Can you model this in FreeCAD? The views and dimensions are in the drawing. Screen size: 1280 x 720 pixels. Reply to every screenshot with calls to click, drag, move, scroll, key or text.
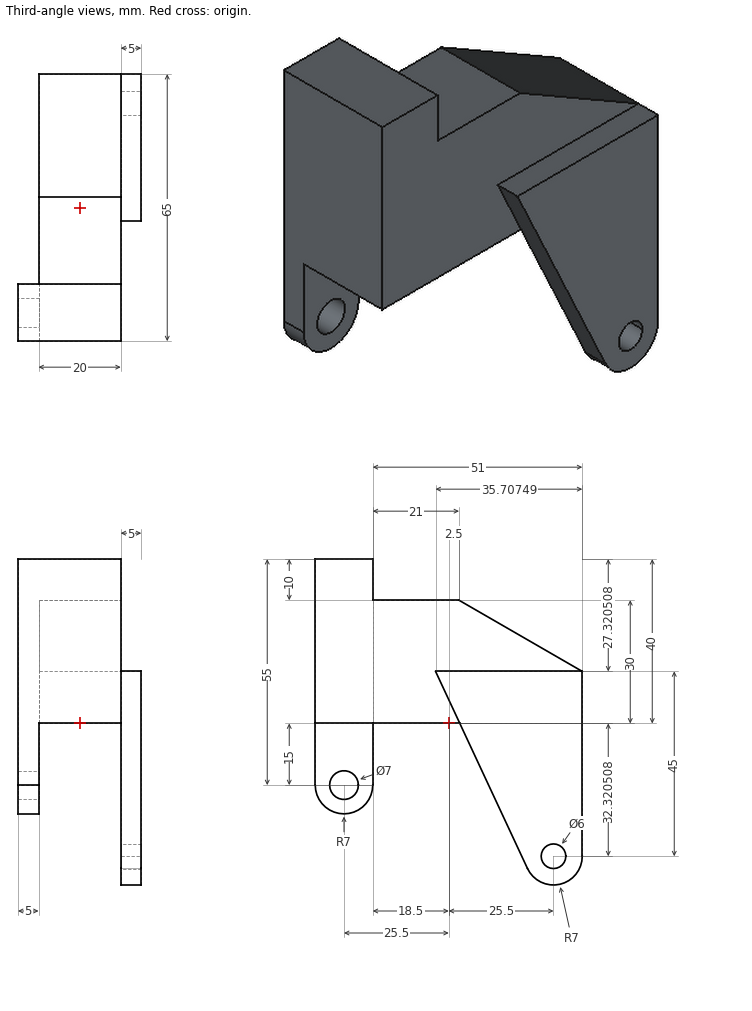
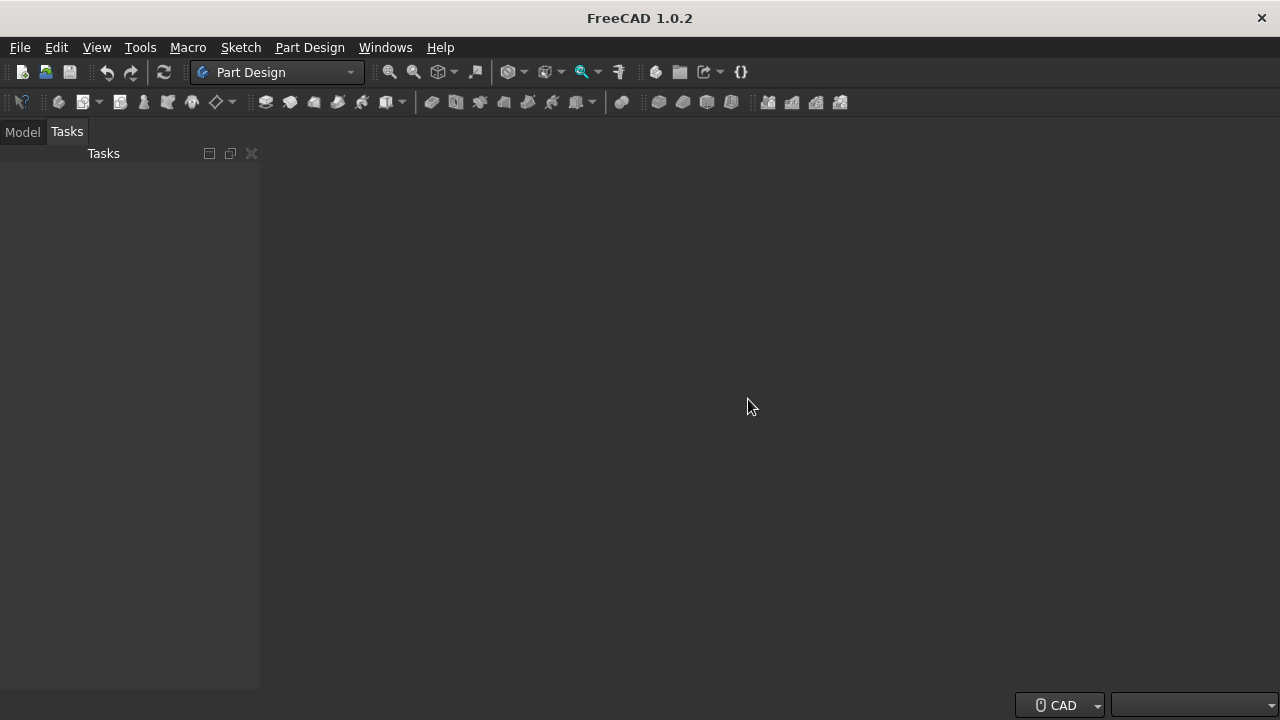
key(ctrl+n)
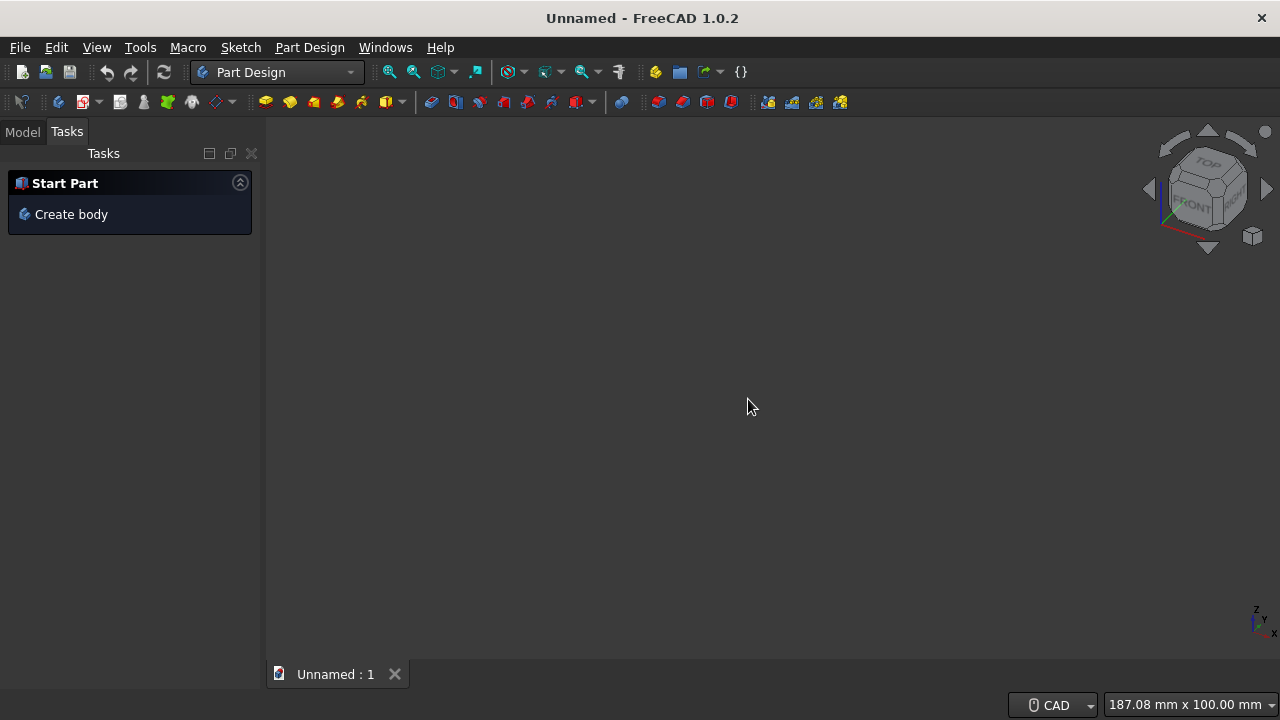
click(84, 102)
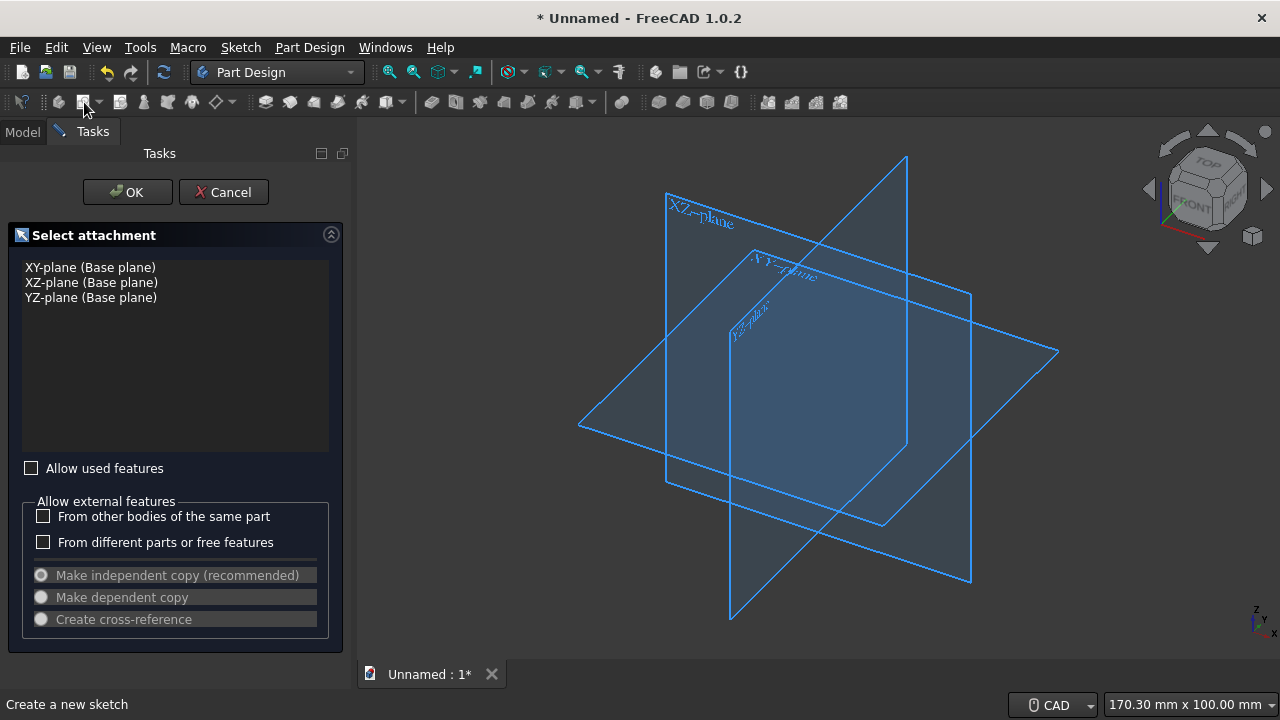
click(82, 268)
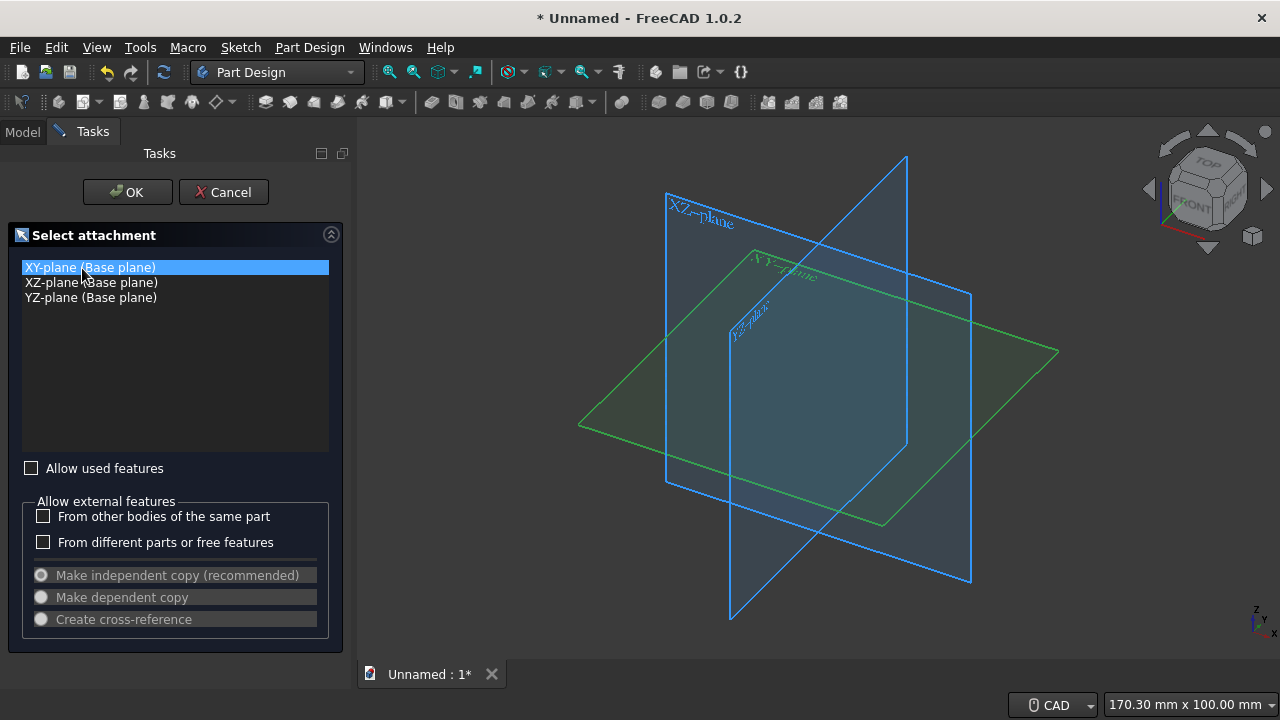
click(128, 192)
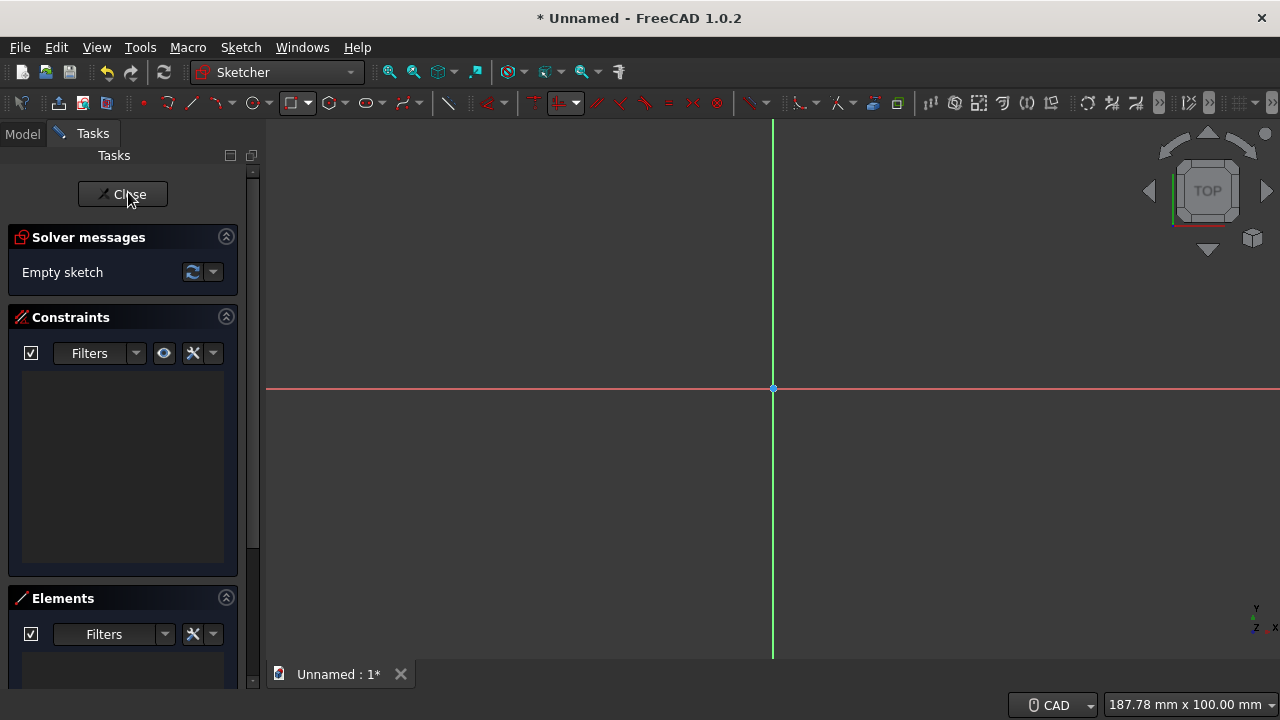
key(g)
key(v)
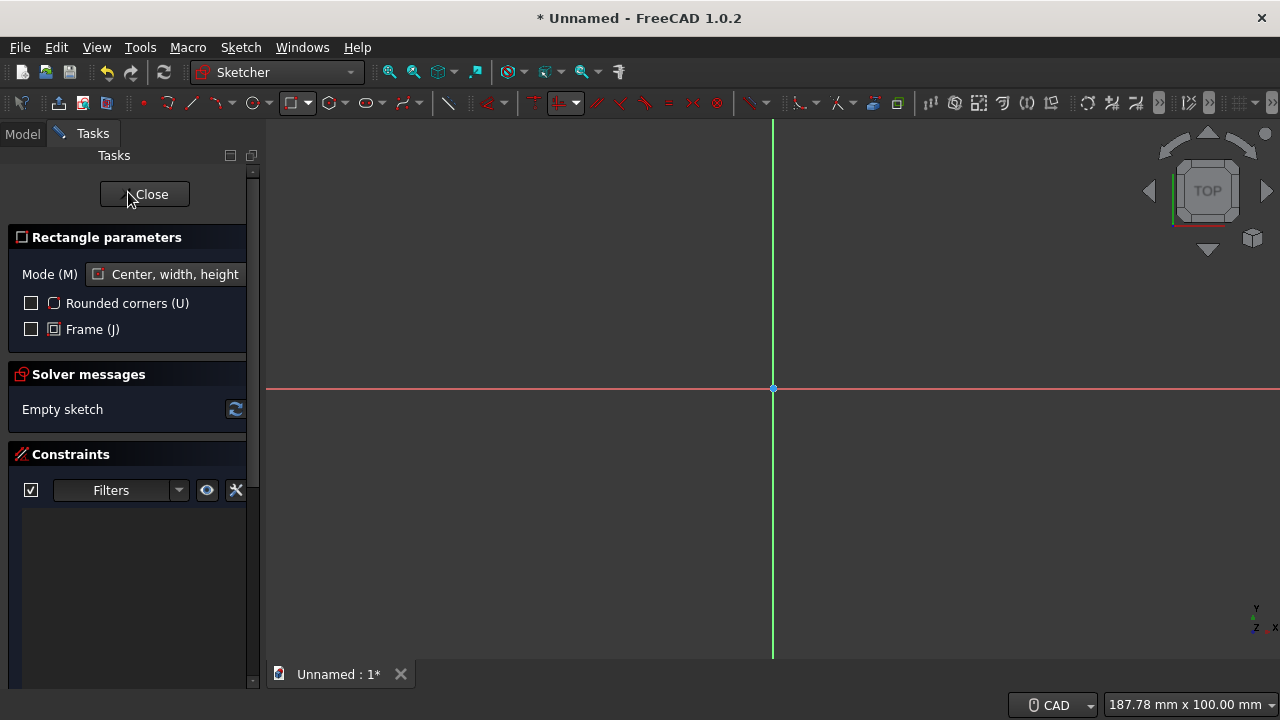
click(773, 389)
move(827, 214)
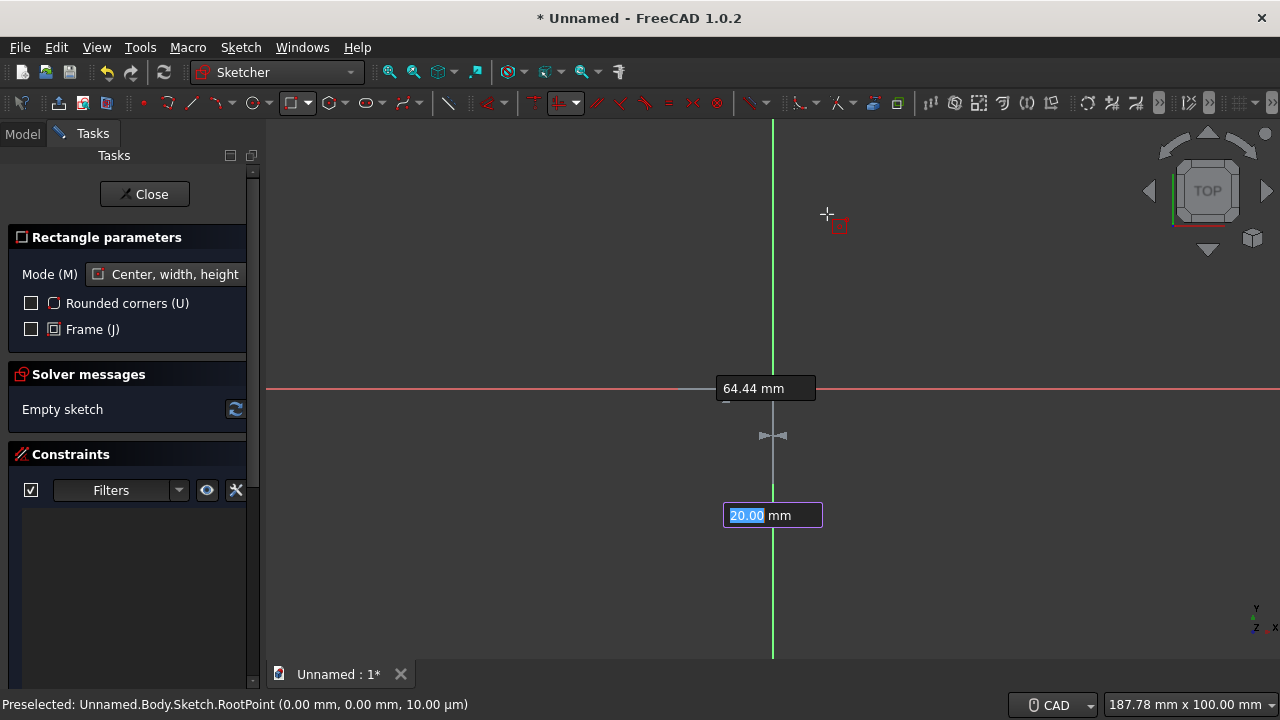
text(20)
key(Tab)
text(65)
key(Return)
key(Escape)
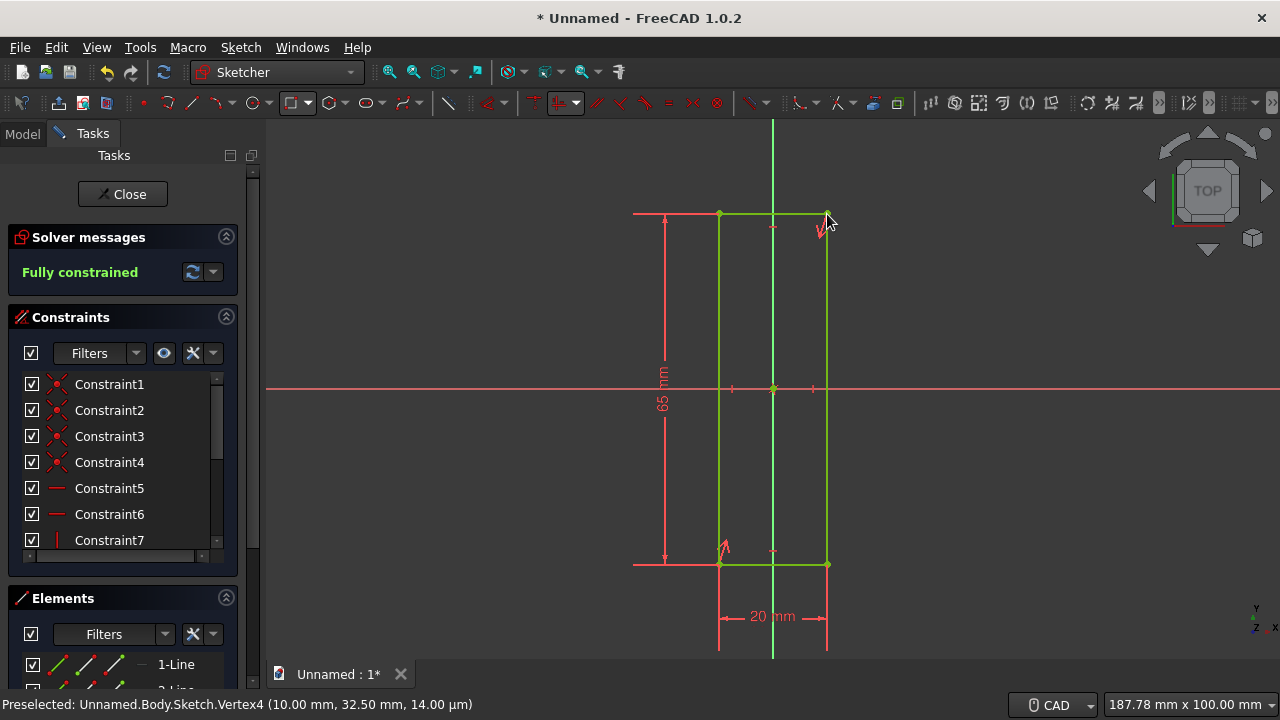
click(123, 194)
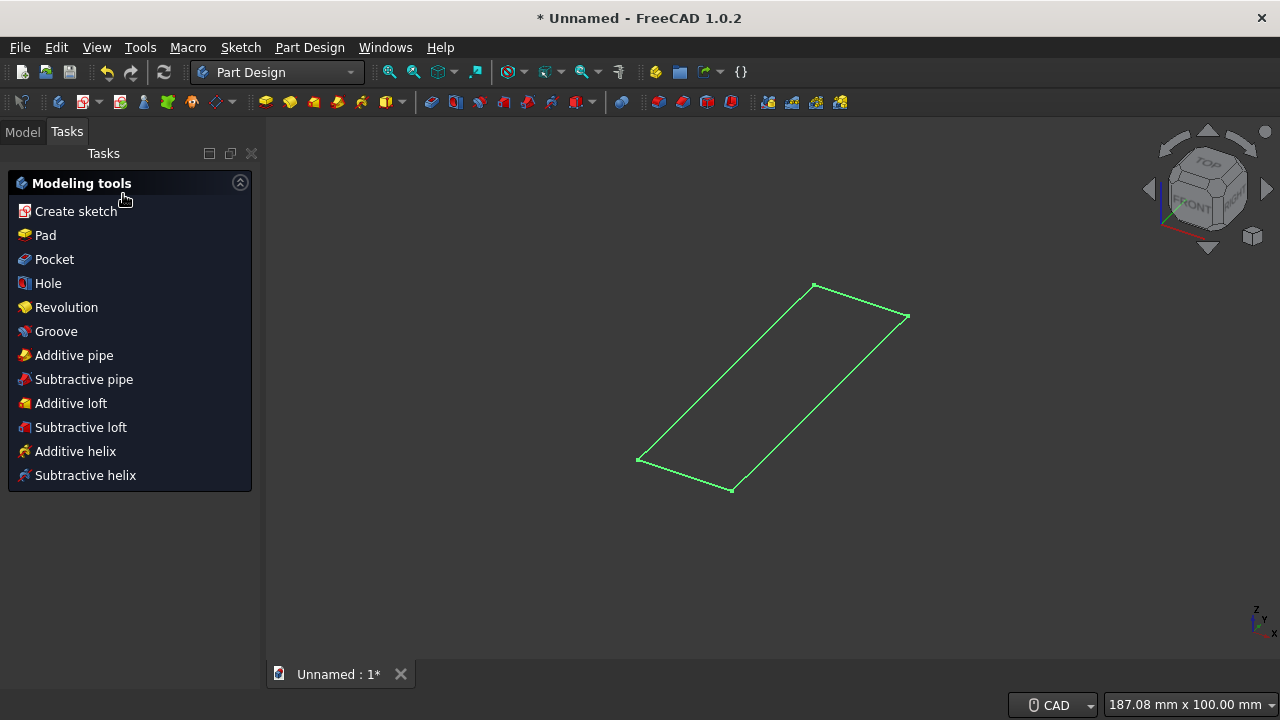
click(266, 102)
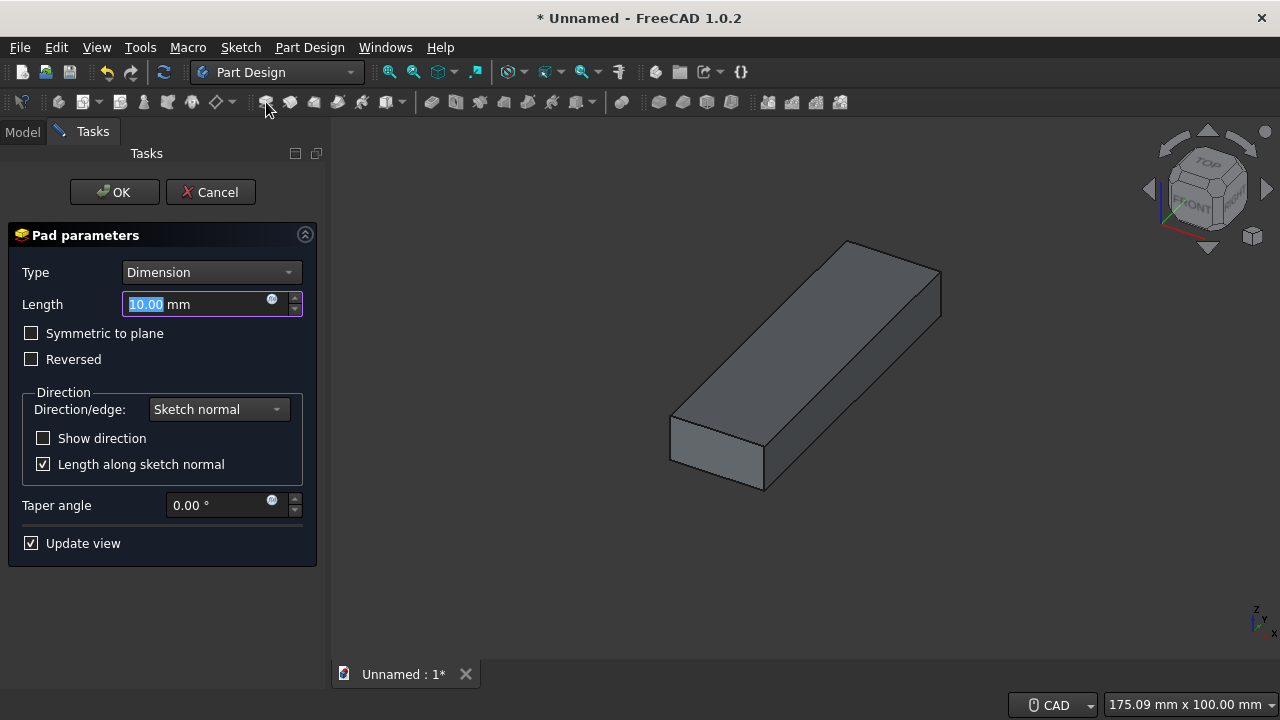
text(40)
key(Tab)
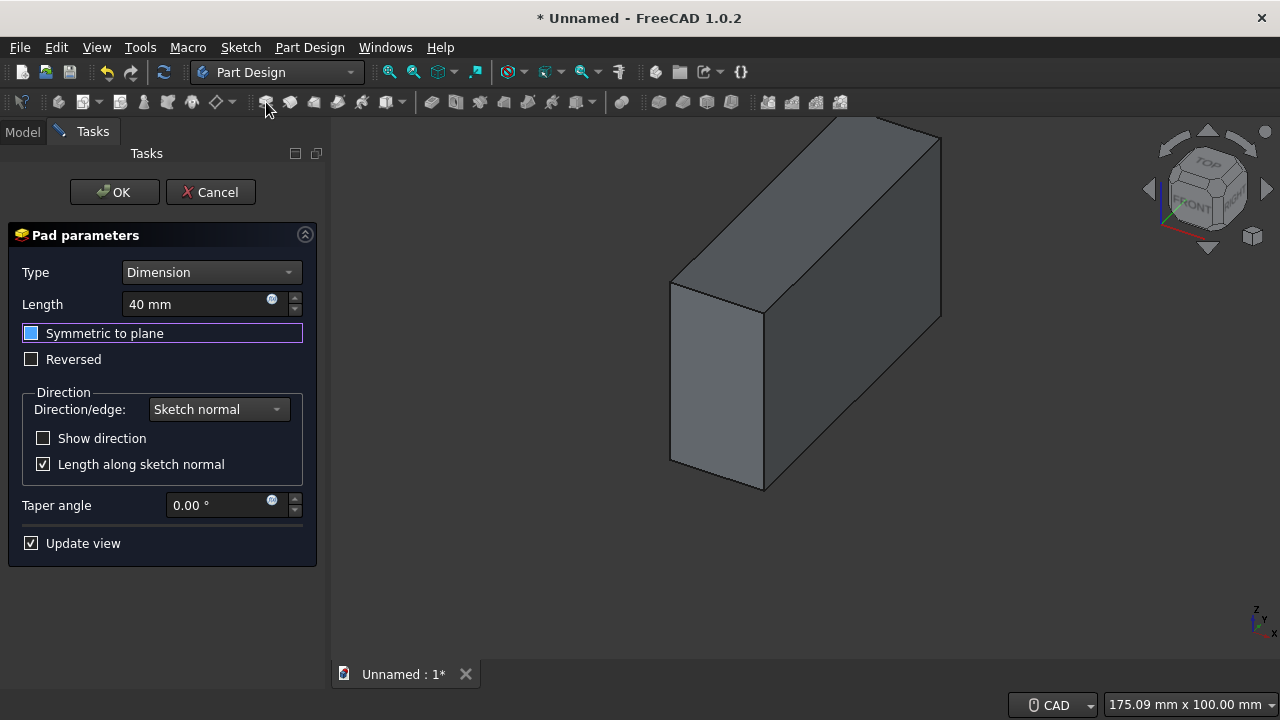
click(115, 192)